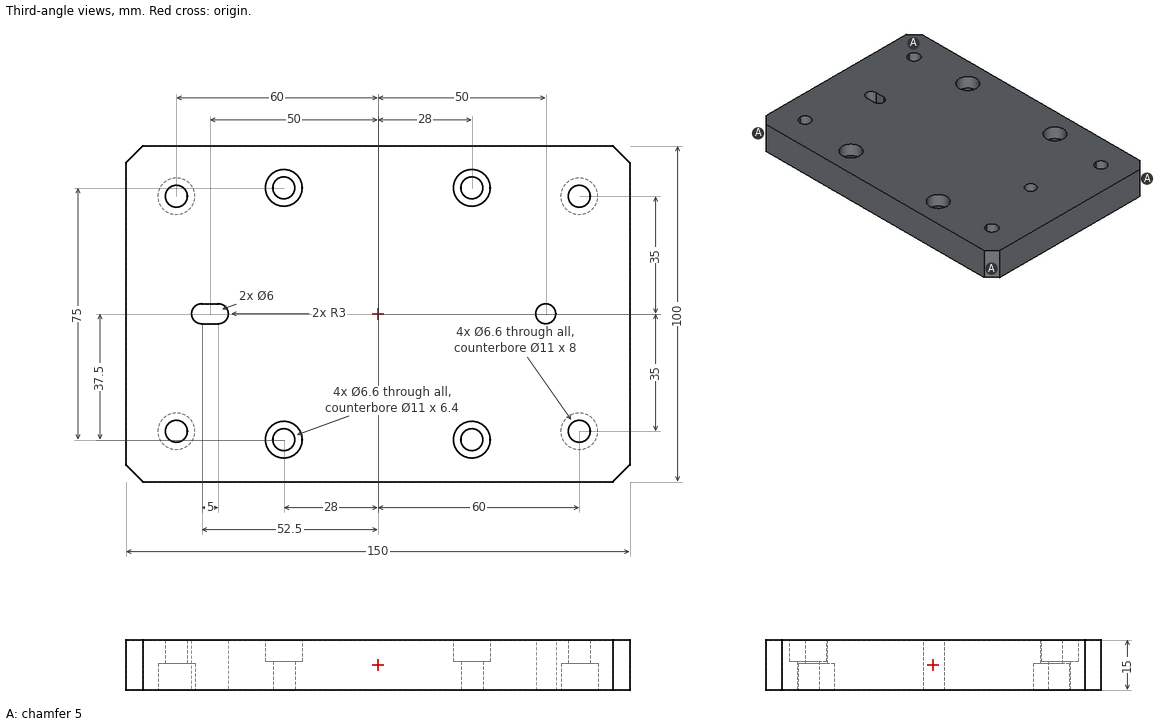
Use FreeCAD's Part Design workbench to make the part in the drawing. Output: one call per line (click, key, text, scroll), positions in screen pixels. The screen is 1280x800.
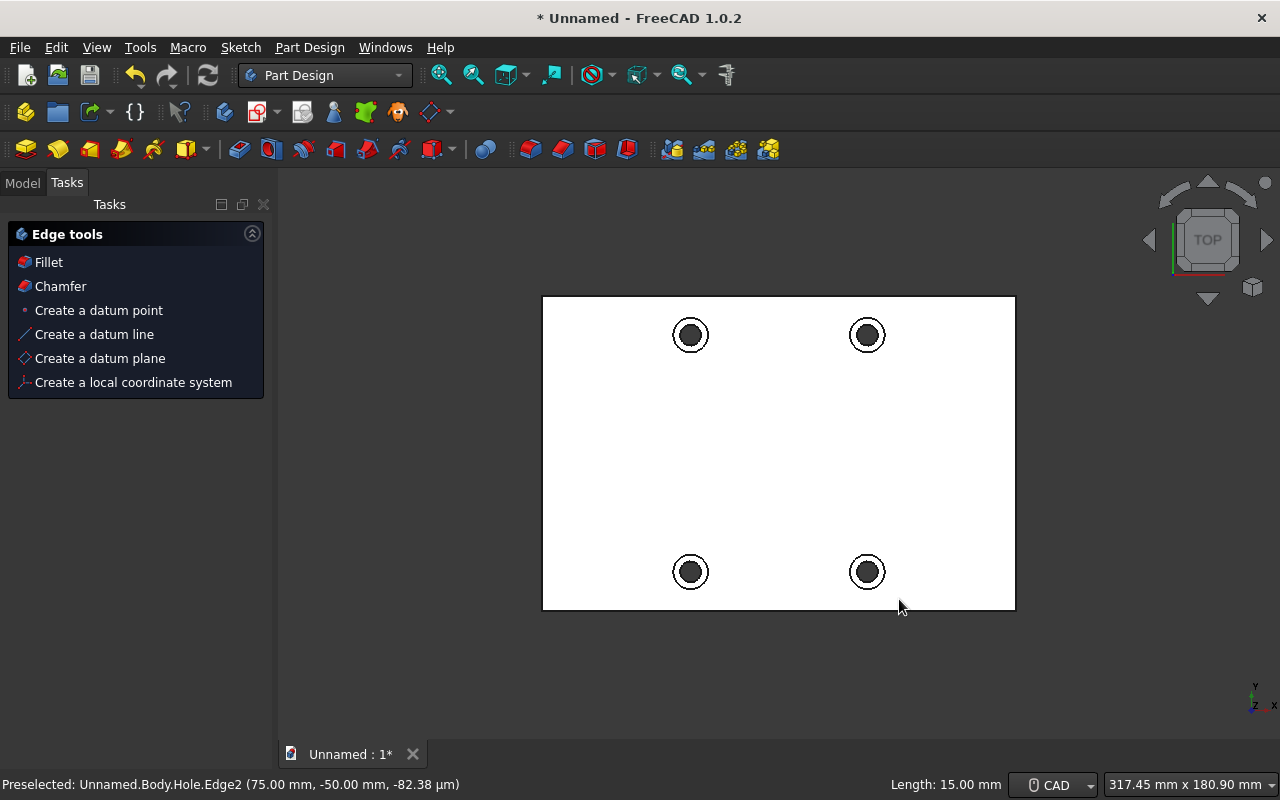
key(1)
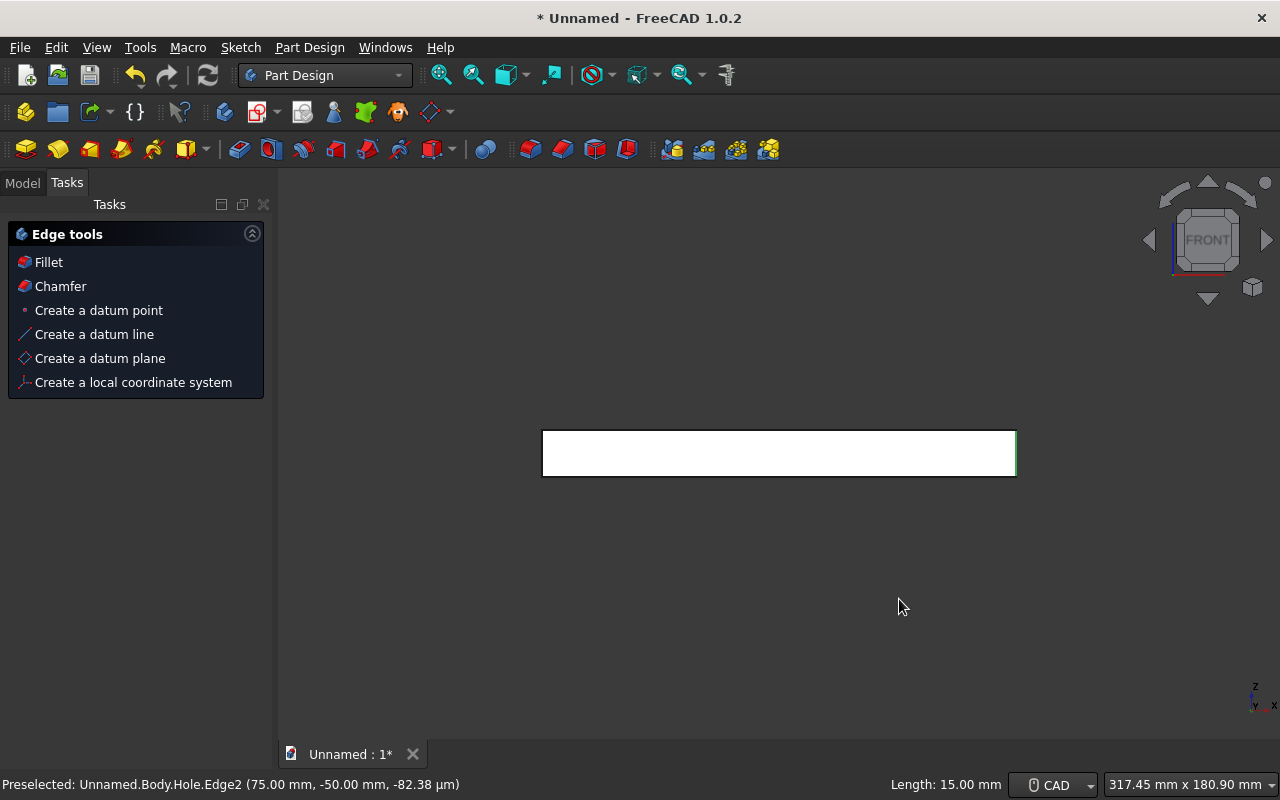
click(542, 452, ctrl)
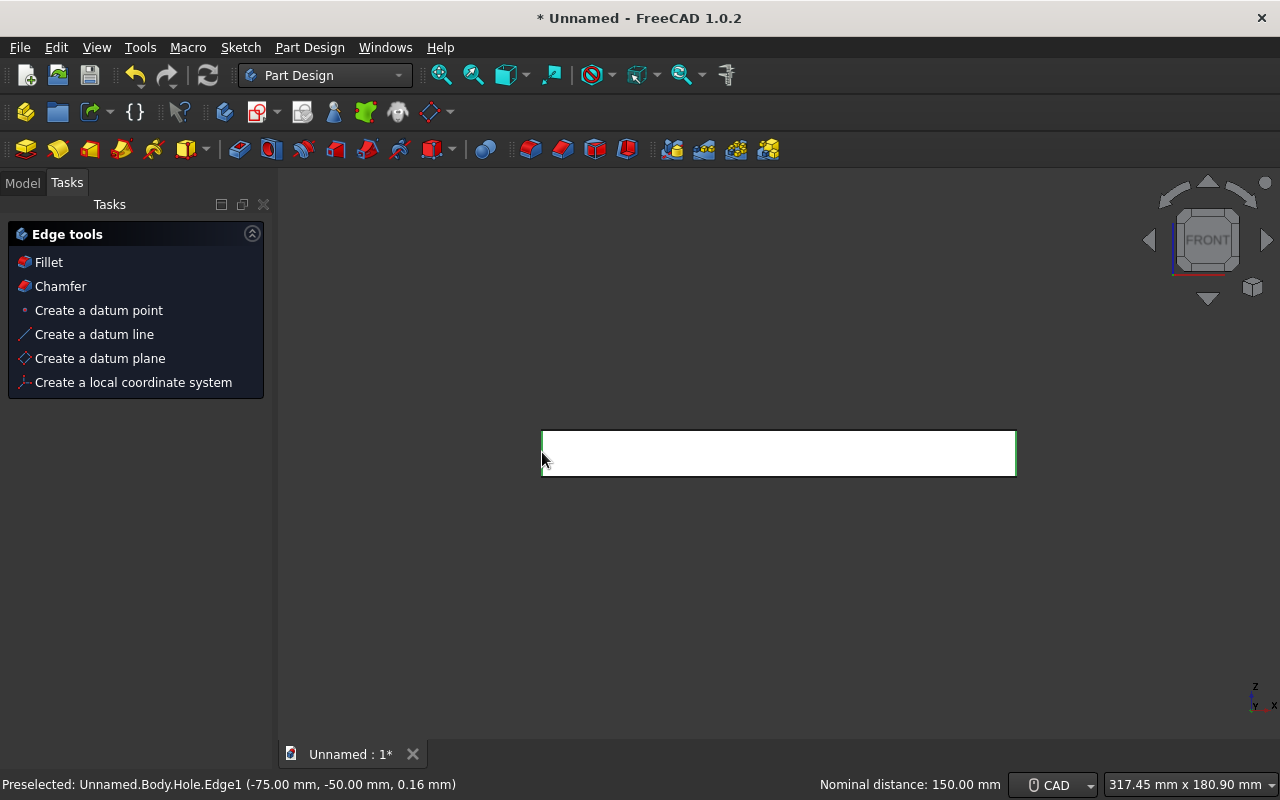
key(3)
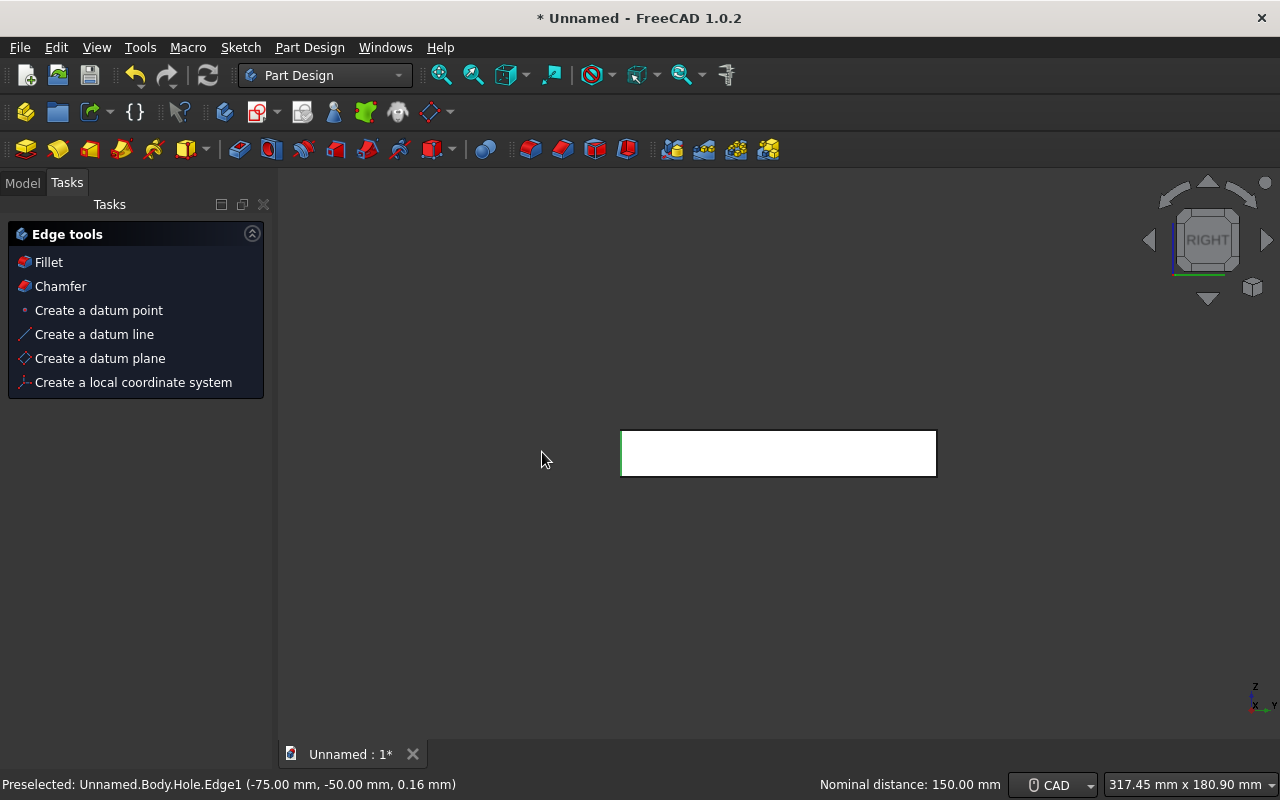
key(v)
key(f)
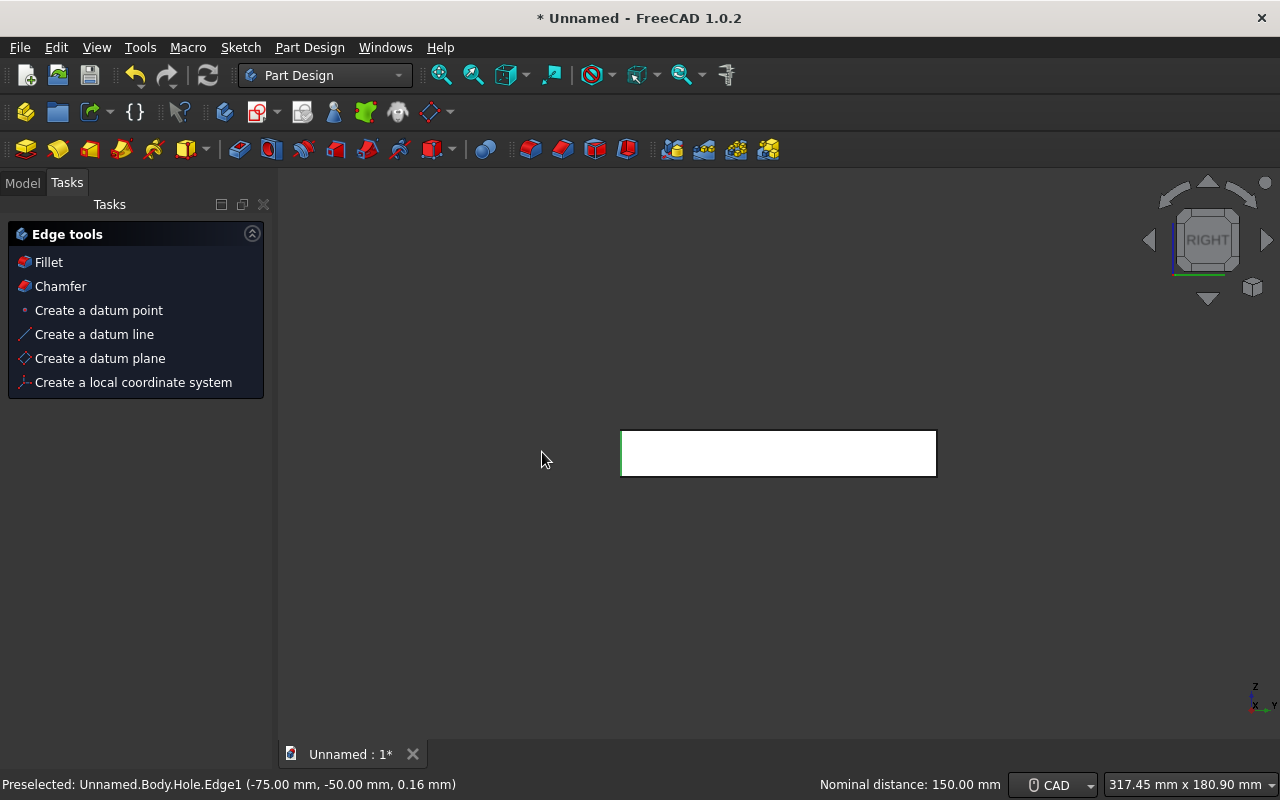
click(937, 452, ctrl)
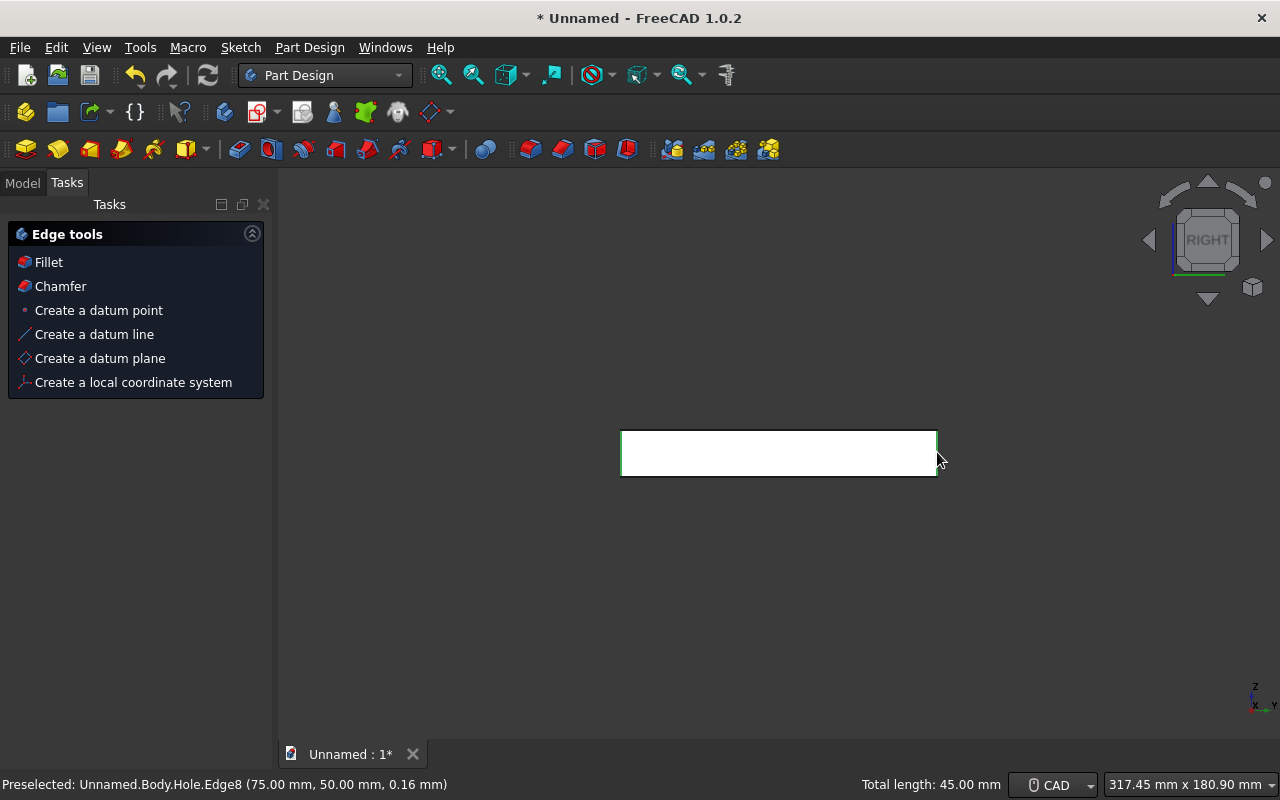
key(5)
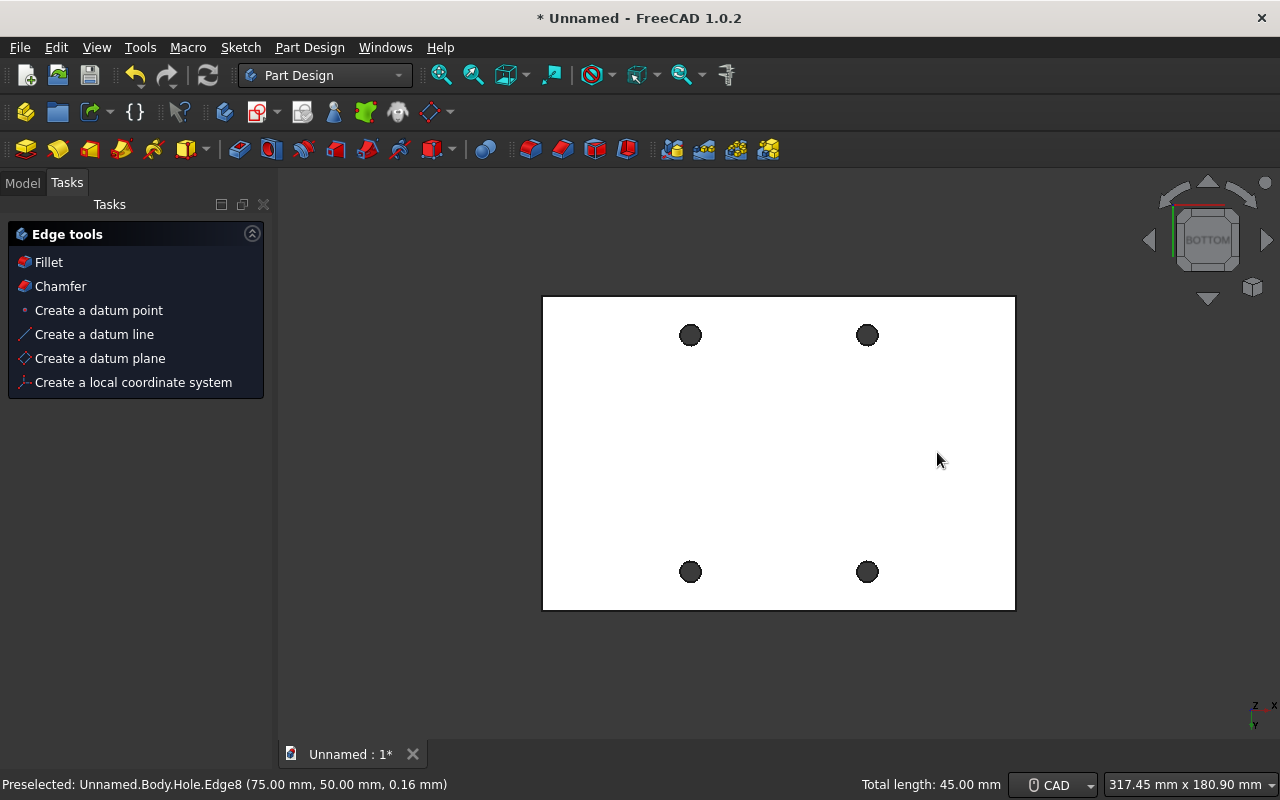
key(4)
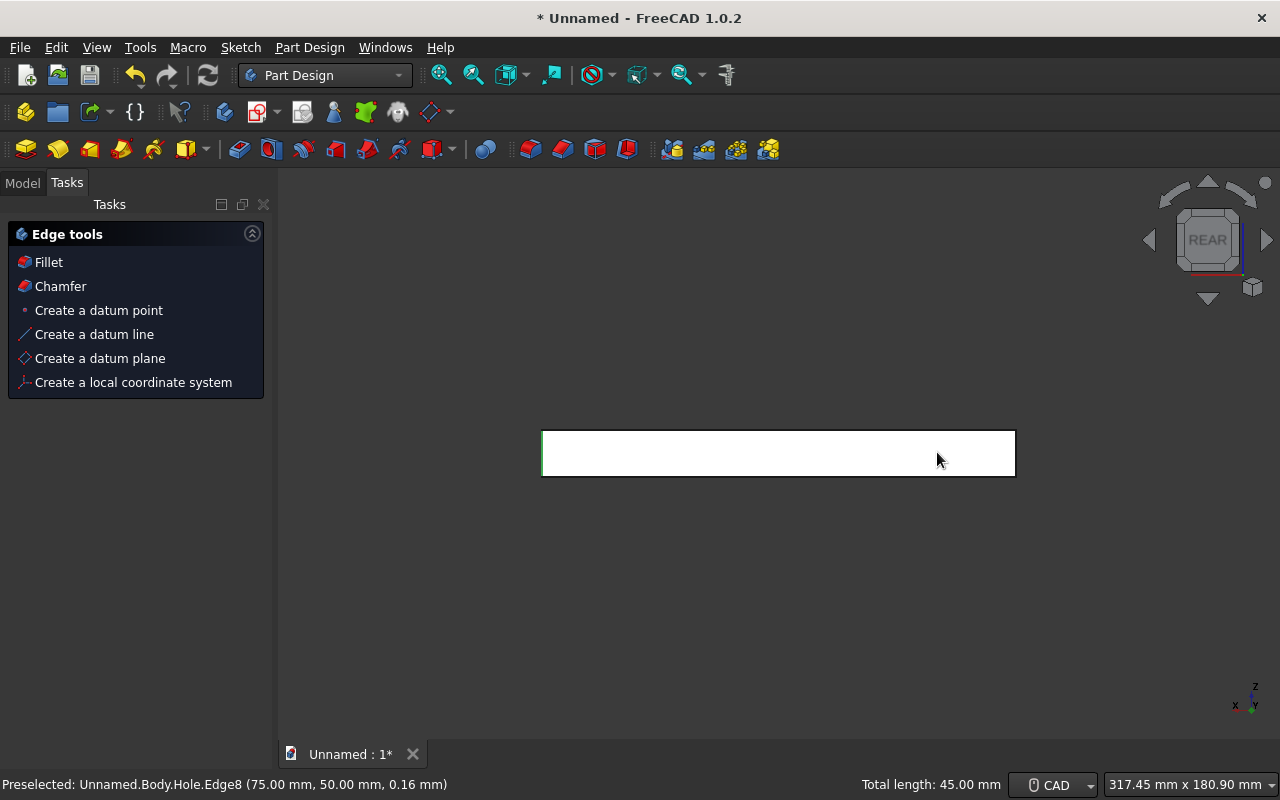
click(1016, 453, ctrl)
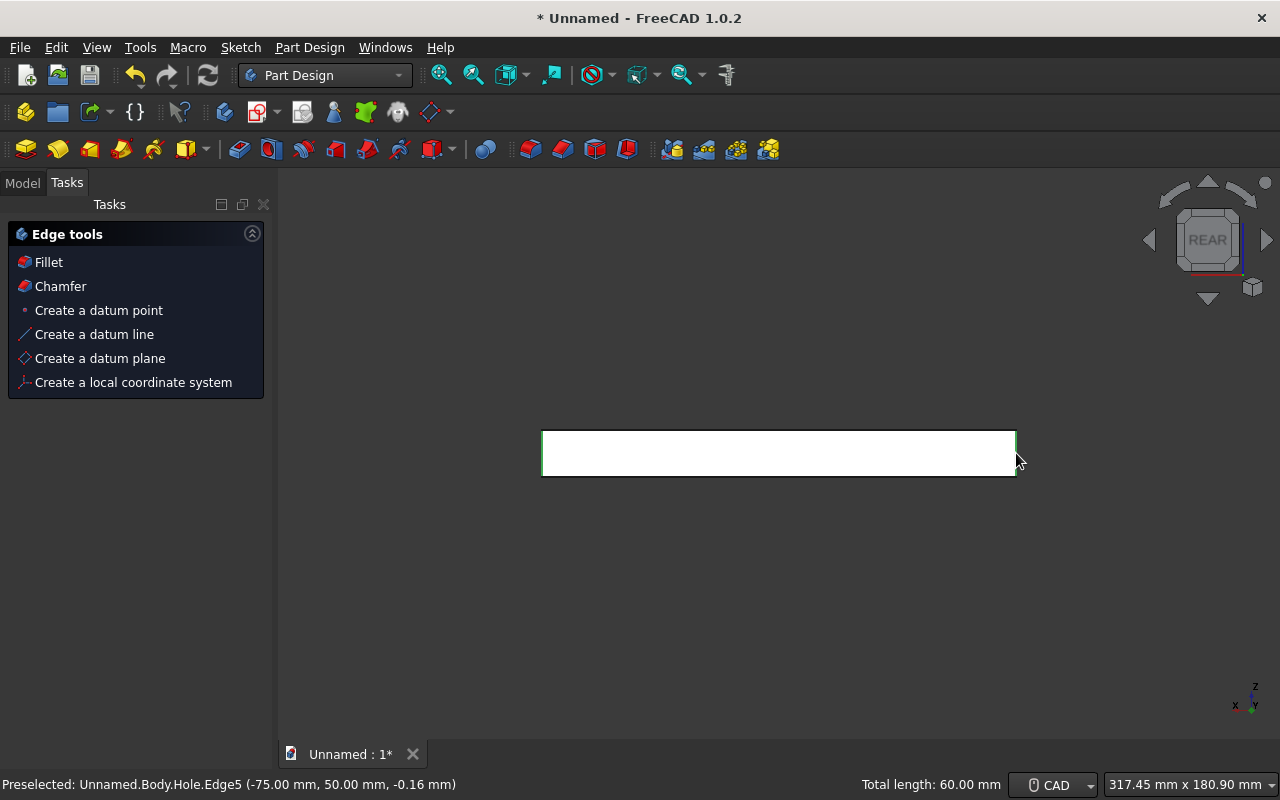
click(564, 150)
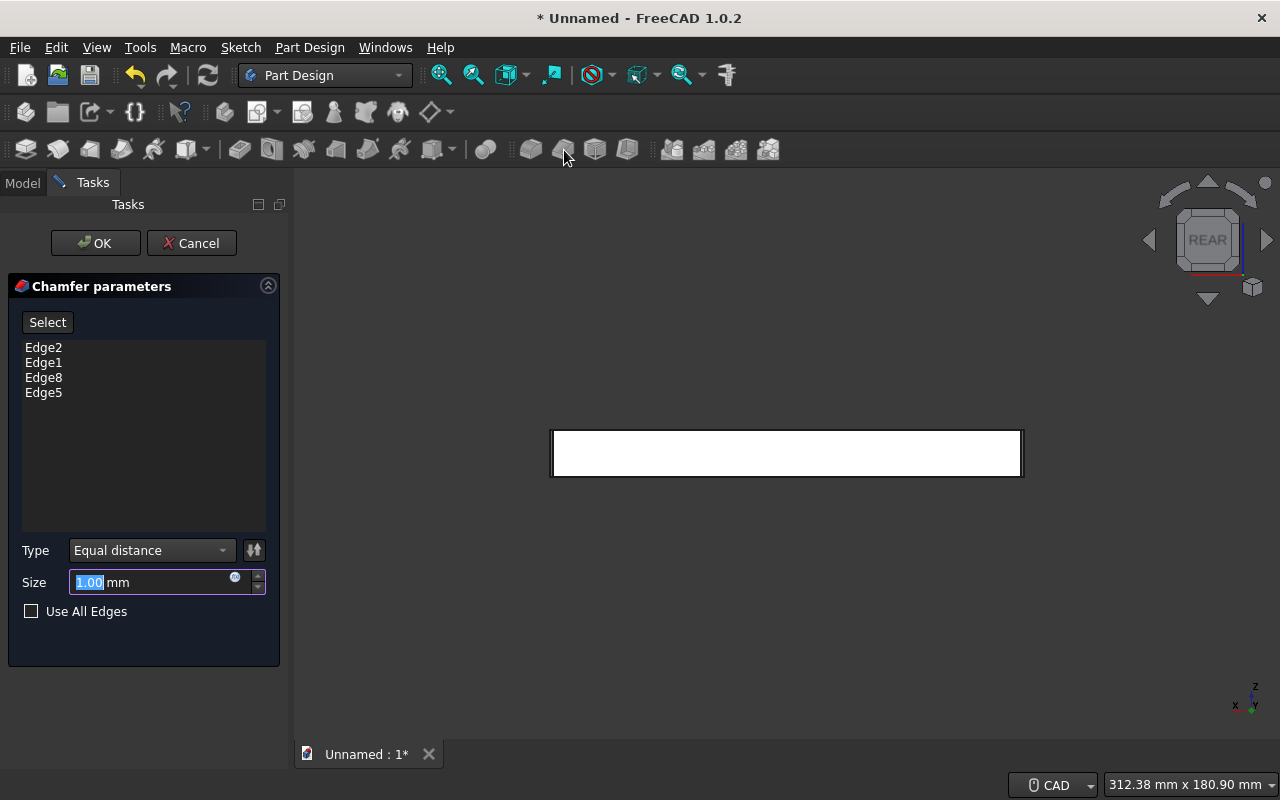
text(5)
key(Tab)